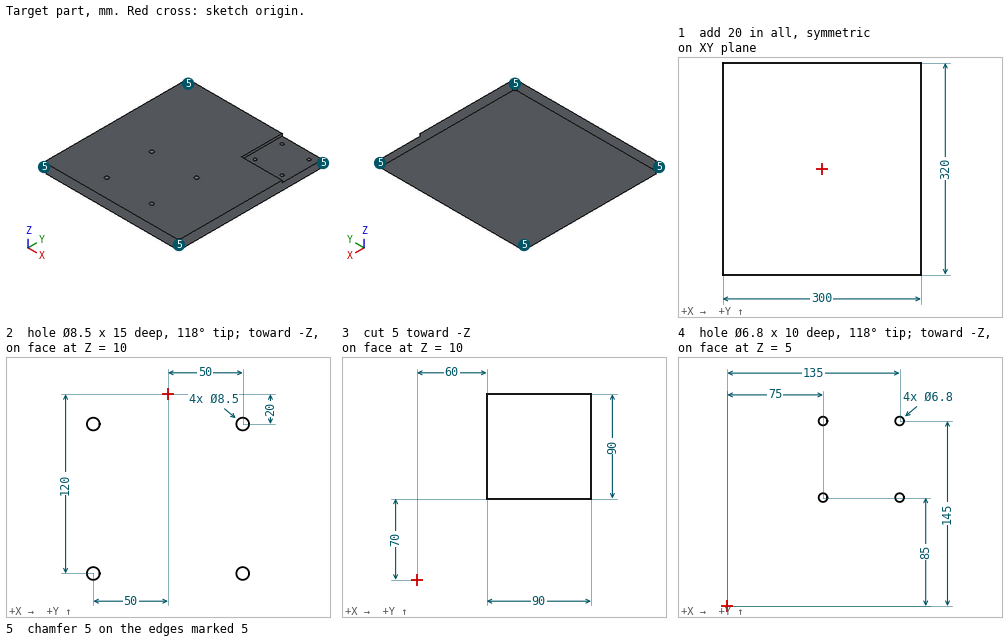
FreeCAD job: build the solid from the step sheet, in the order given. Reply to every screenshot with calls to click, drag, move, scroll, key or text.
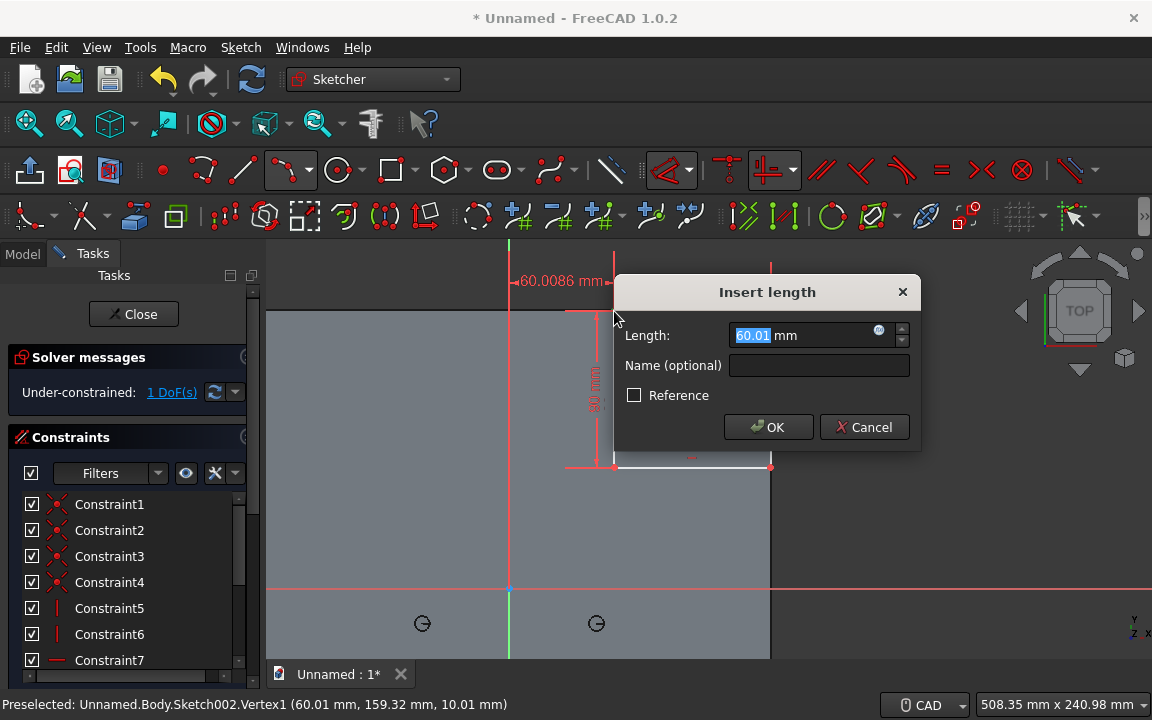
text(60)
key(Return)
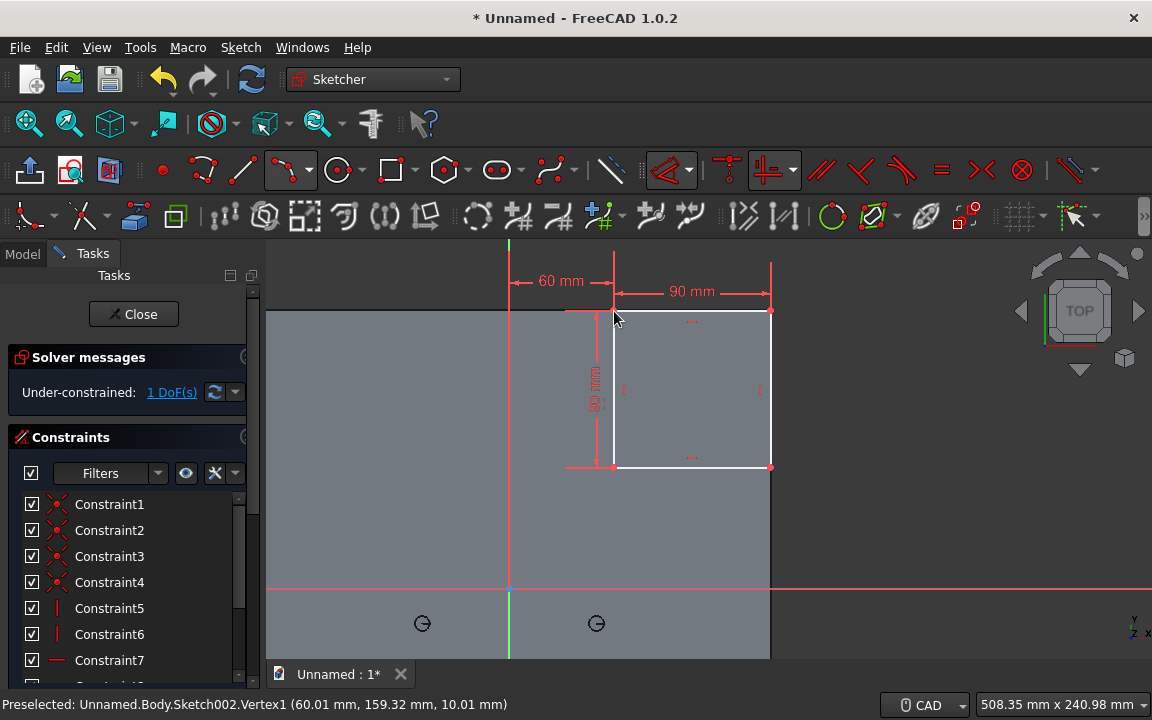
click(614, 468)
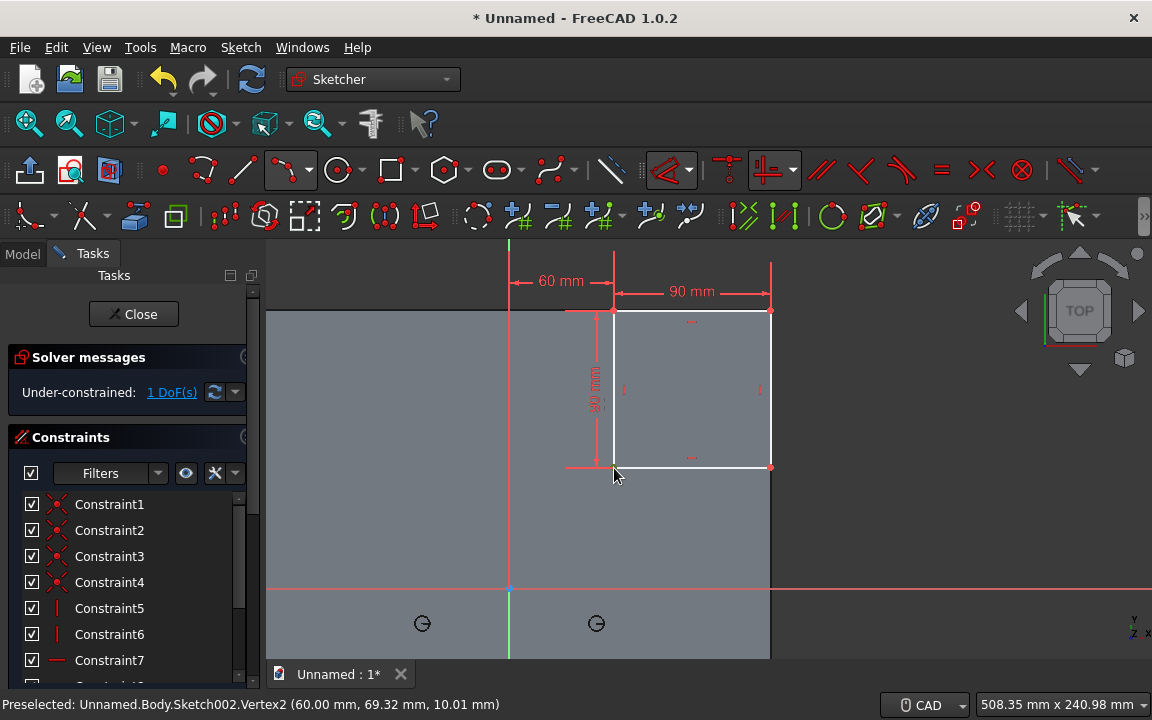
click(692, 170)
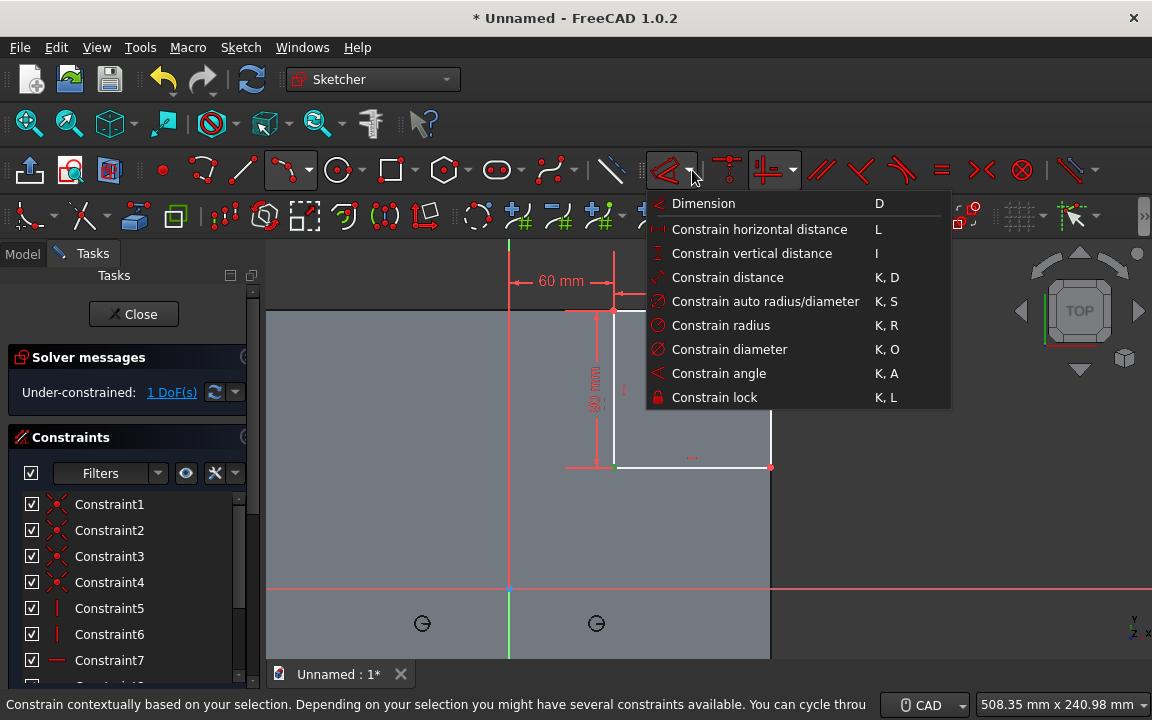
click(799, 253)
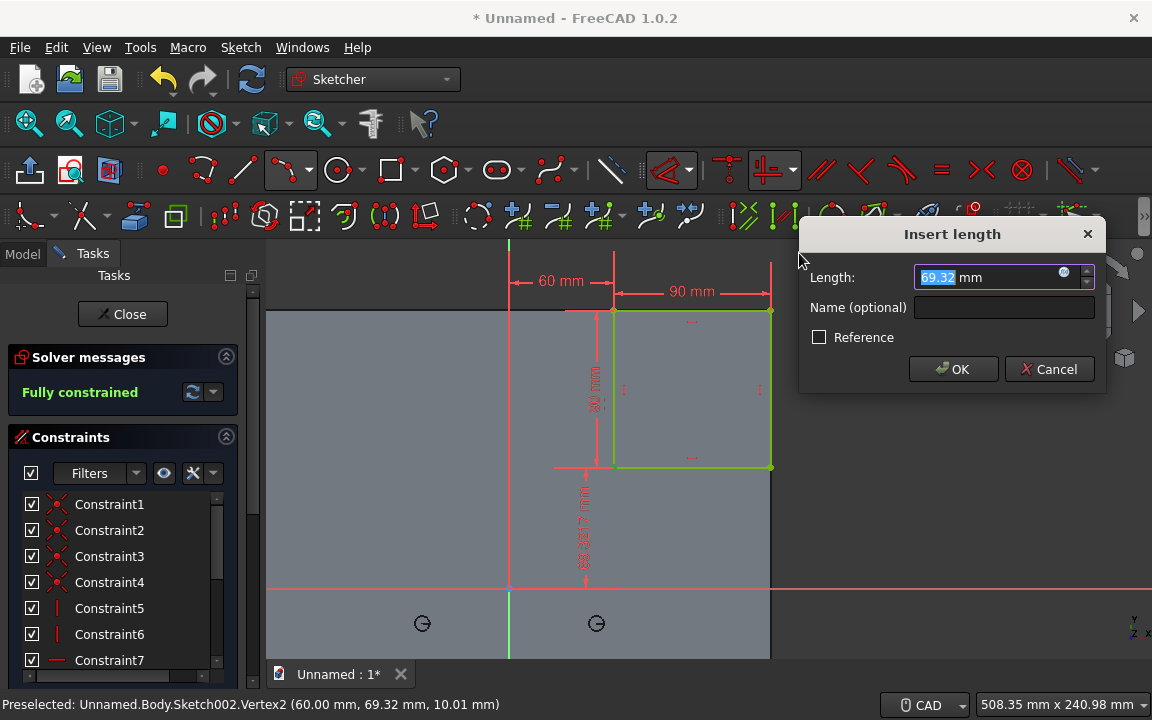
text(70)
key(Return)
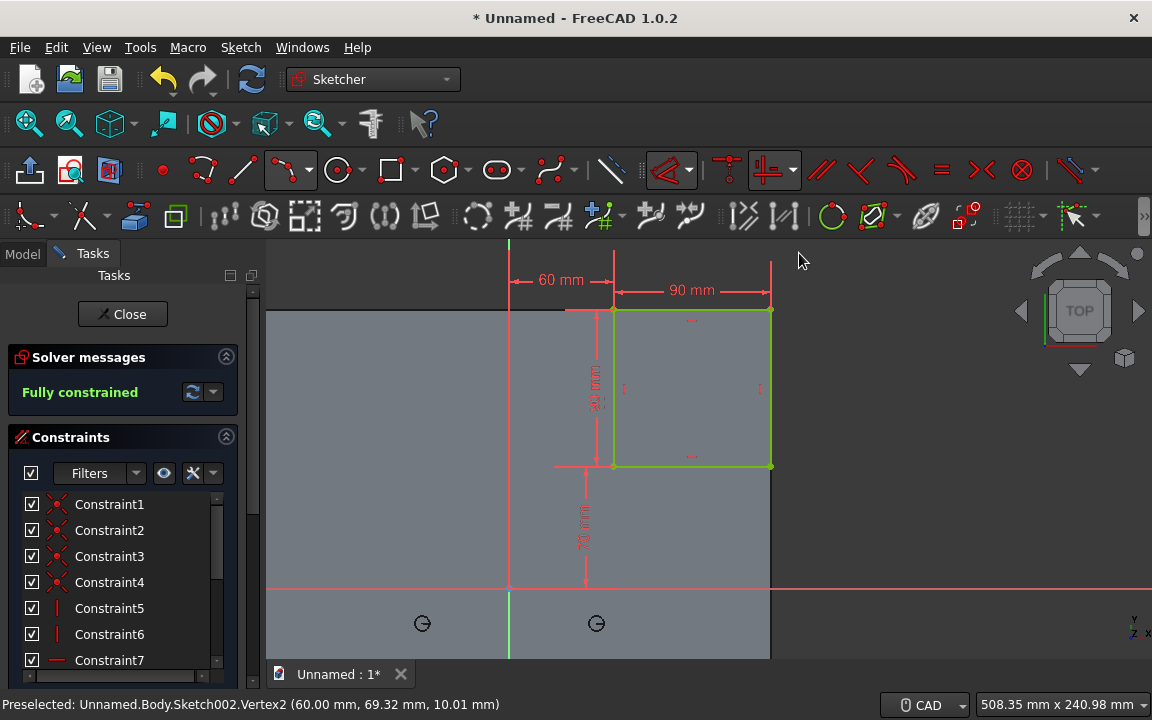
click(123, 314)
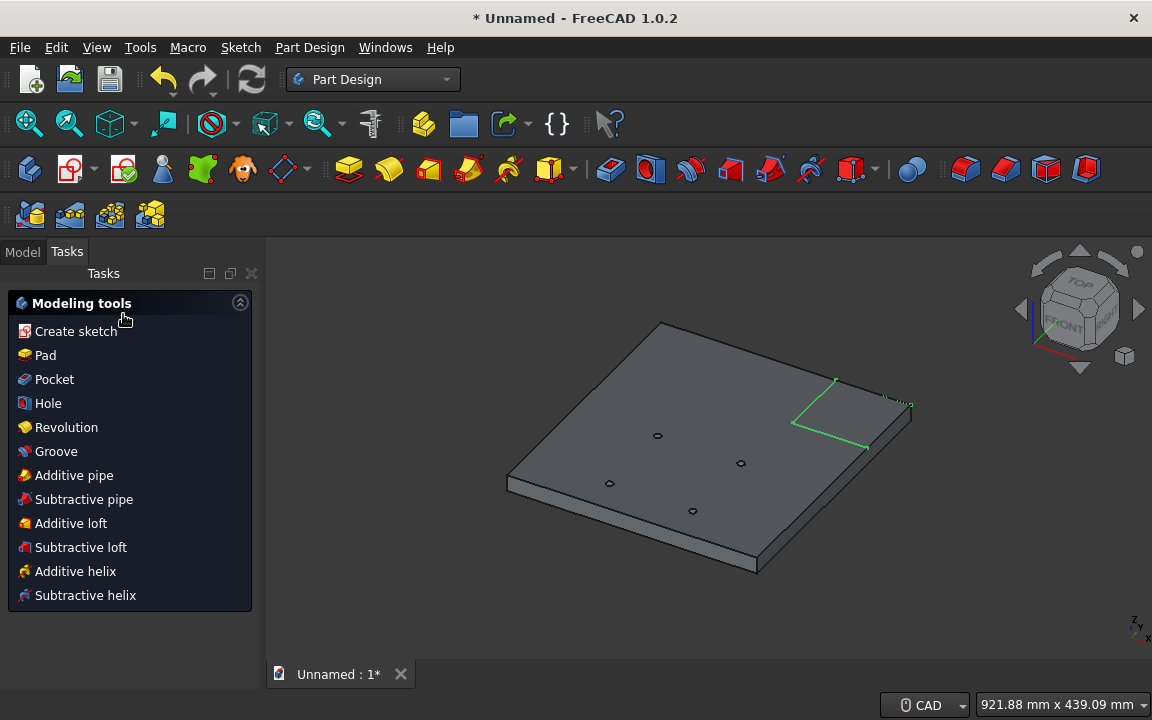
click(612, 170)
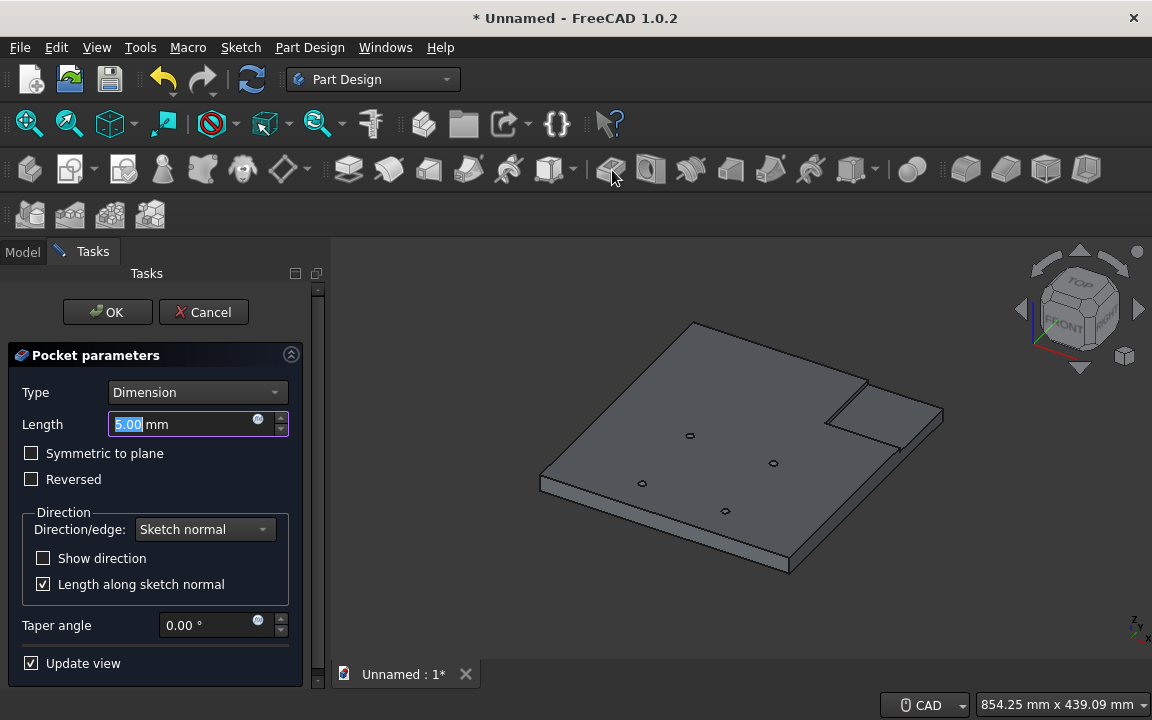
text(5)
key(Tab)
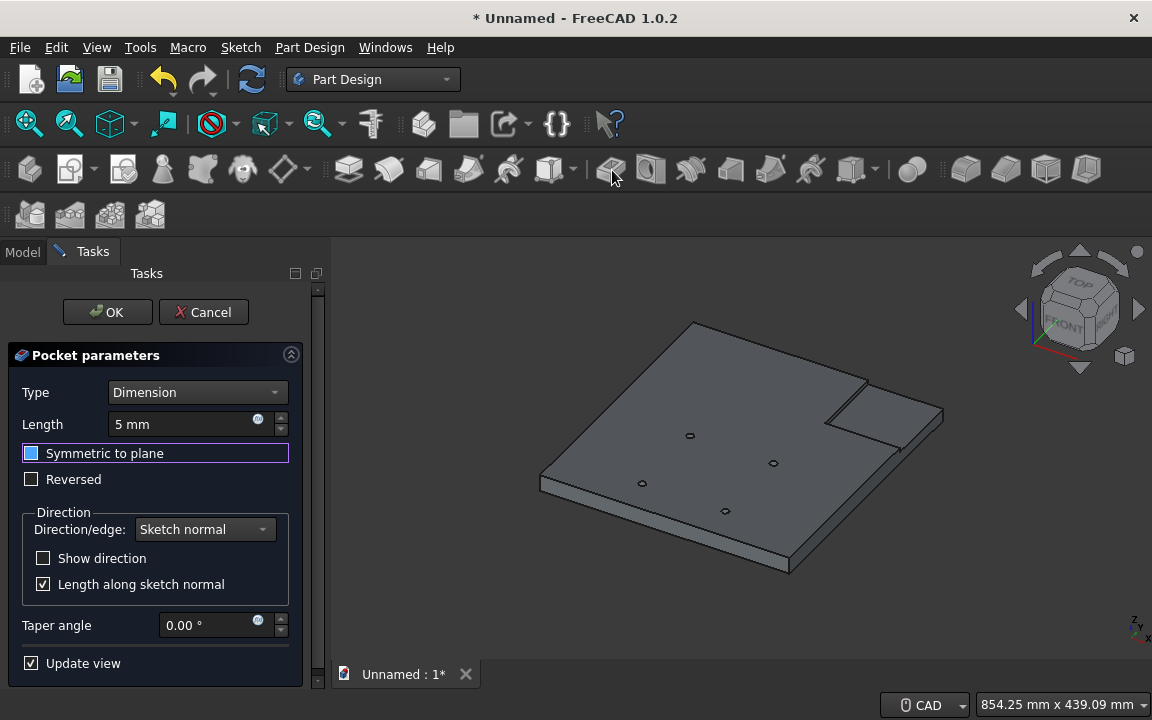
click(108, 312)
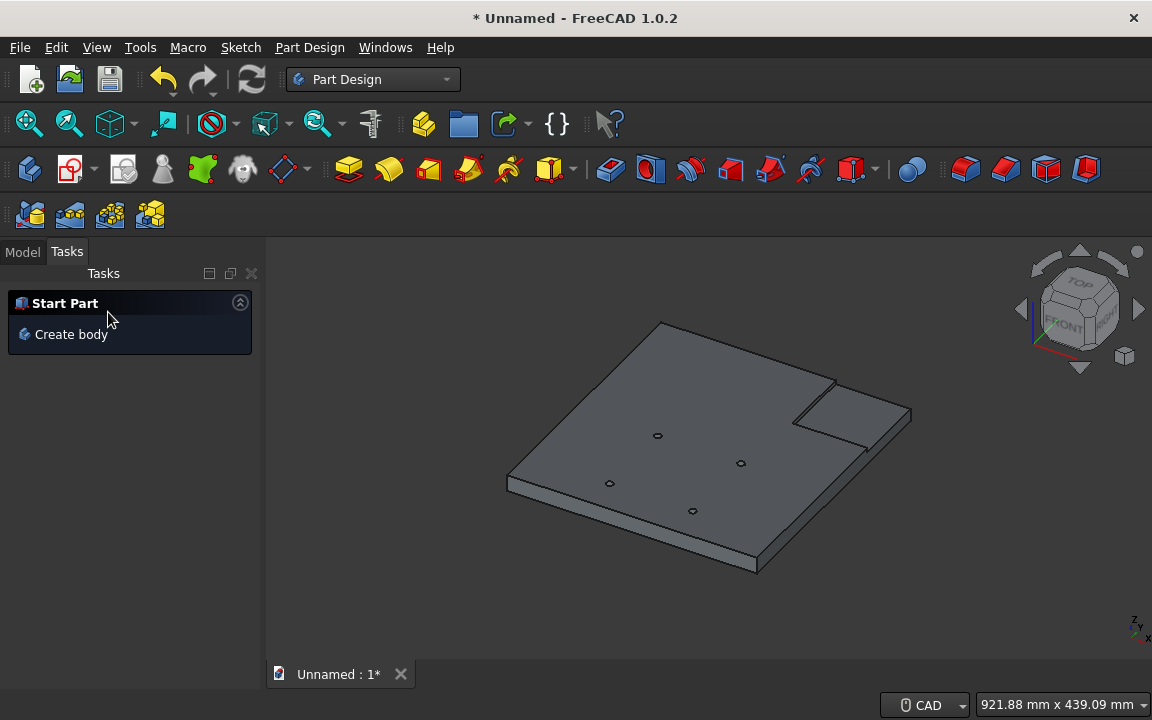
click(852, 417)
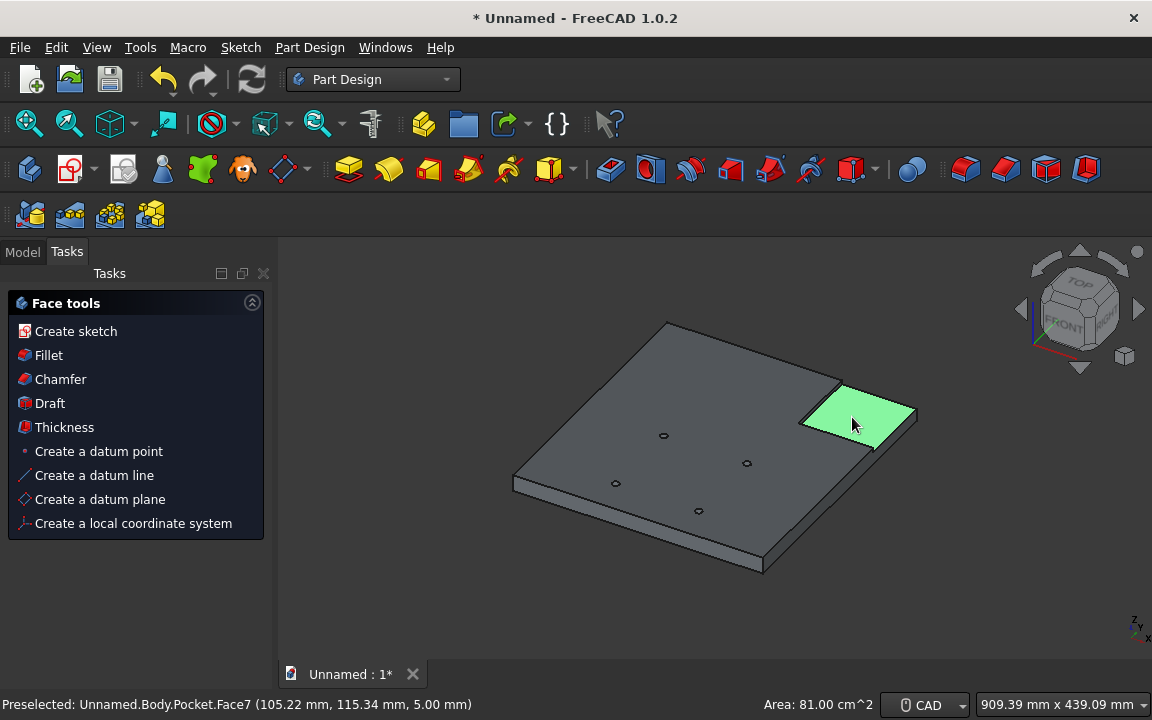
click(70, 170)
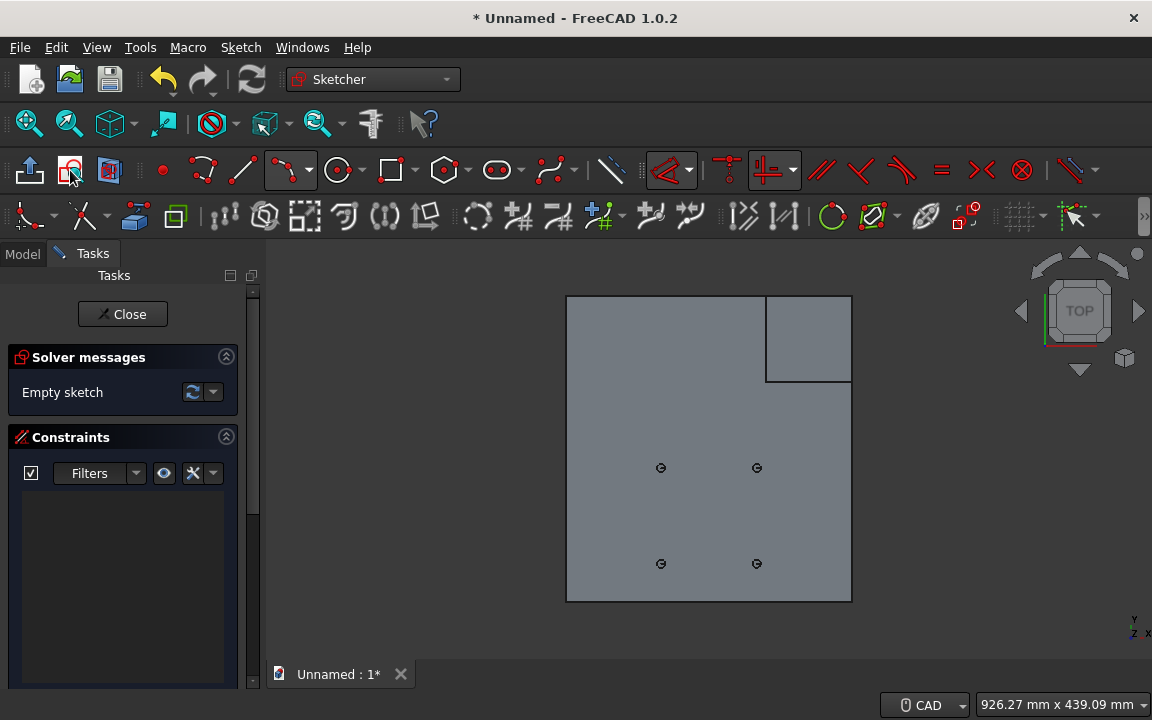
key(q)
key(s)